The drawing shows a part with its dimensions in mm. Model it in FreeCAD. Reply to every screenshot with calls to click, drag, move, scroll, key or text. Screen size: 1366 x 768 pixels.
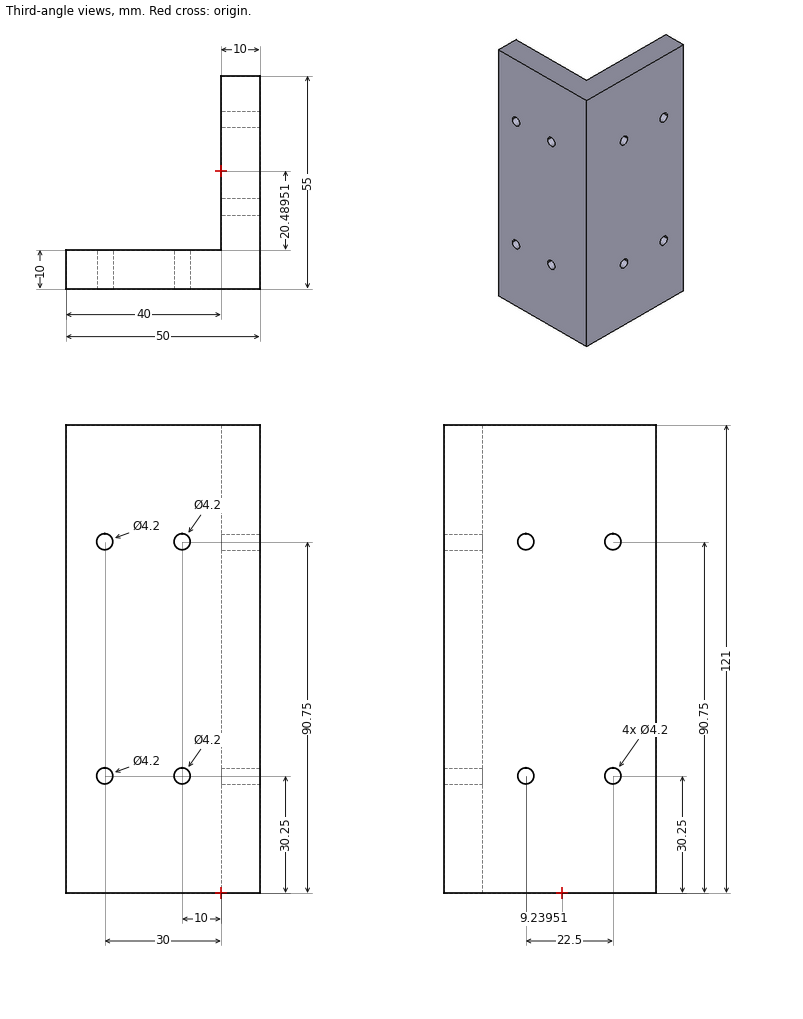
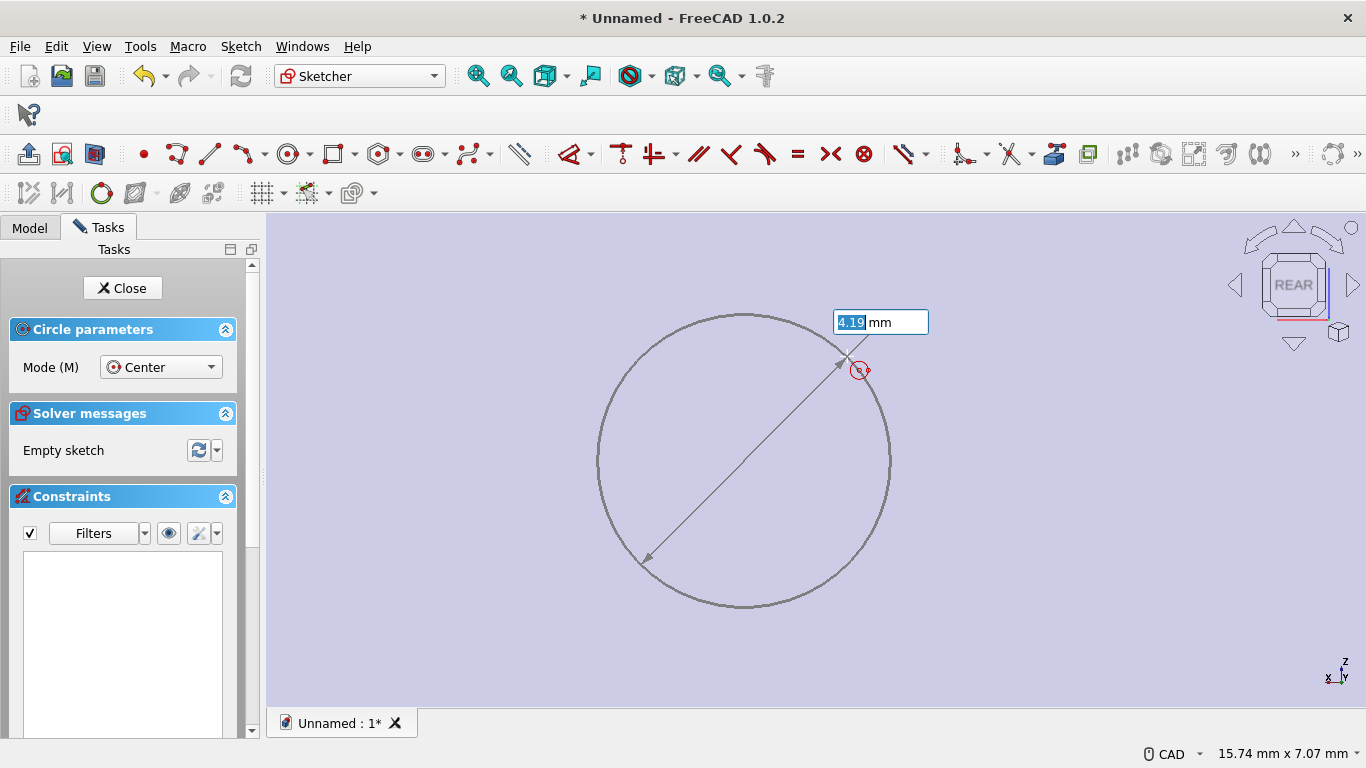
text(4.2)
key(Return)
key(Escape)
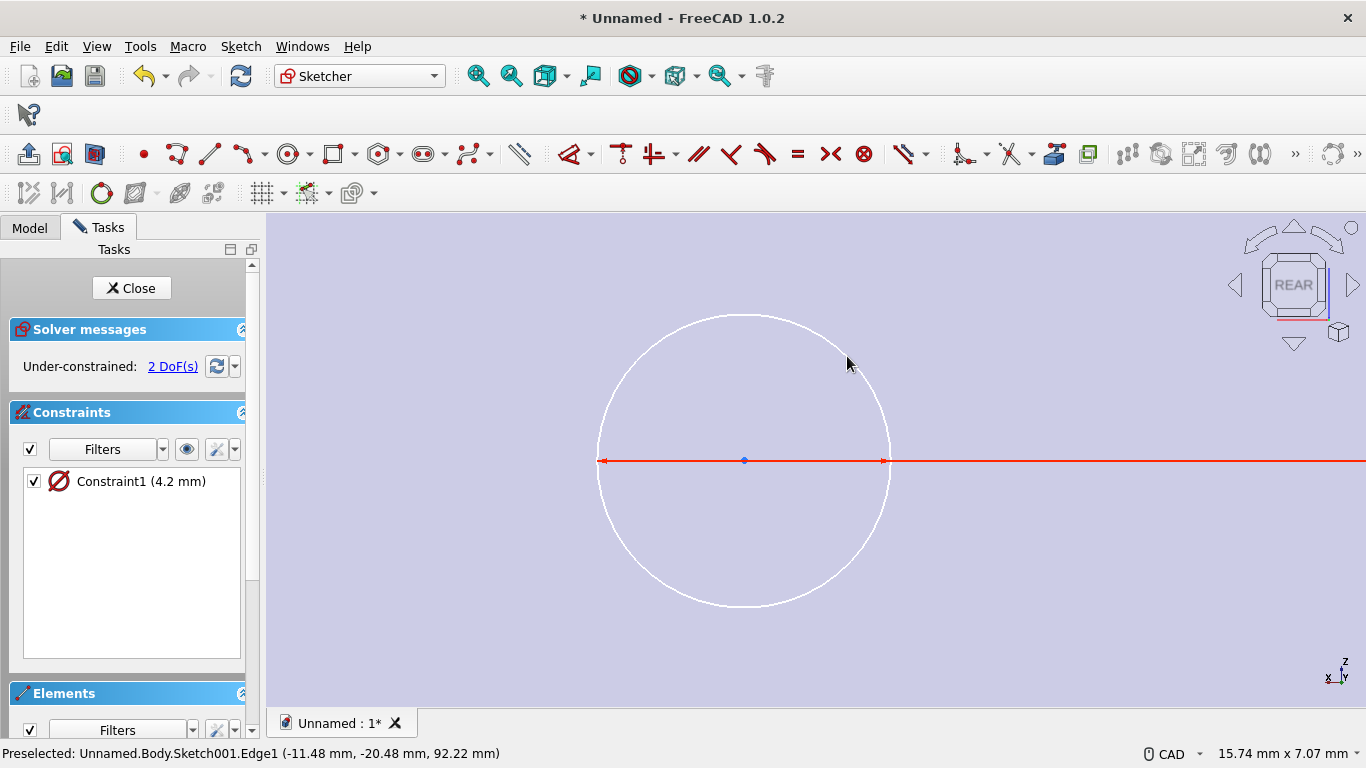
key(d)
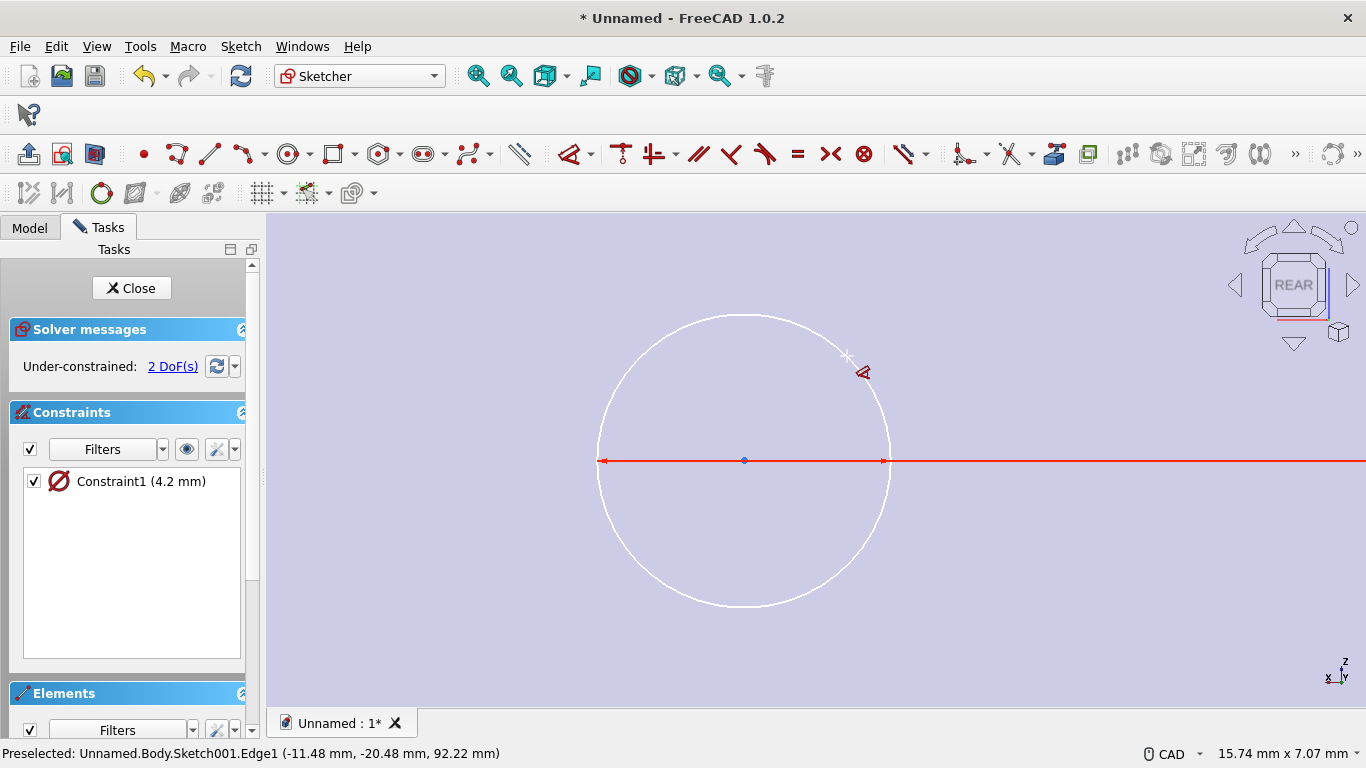
click(744, 461)
click(519, 427)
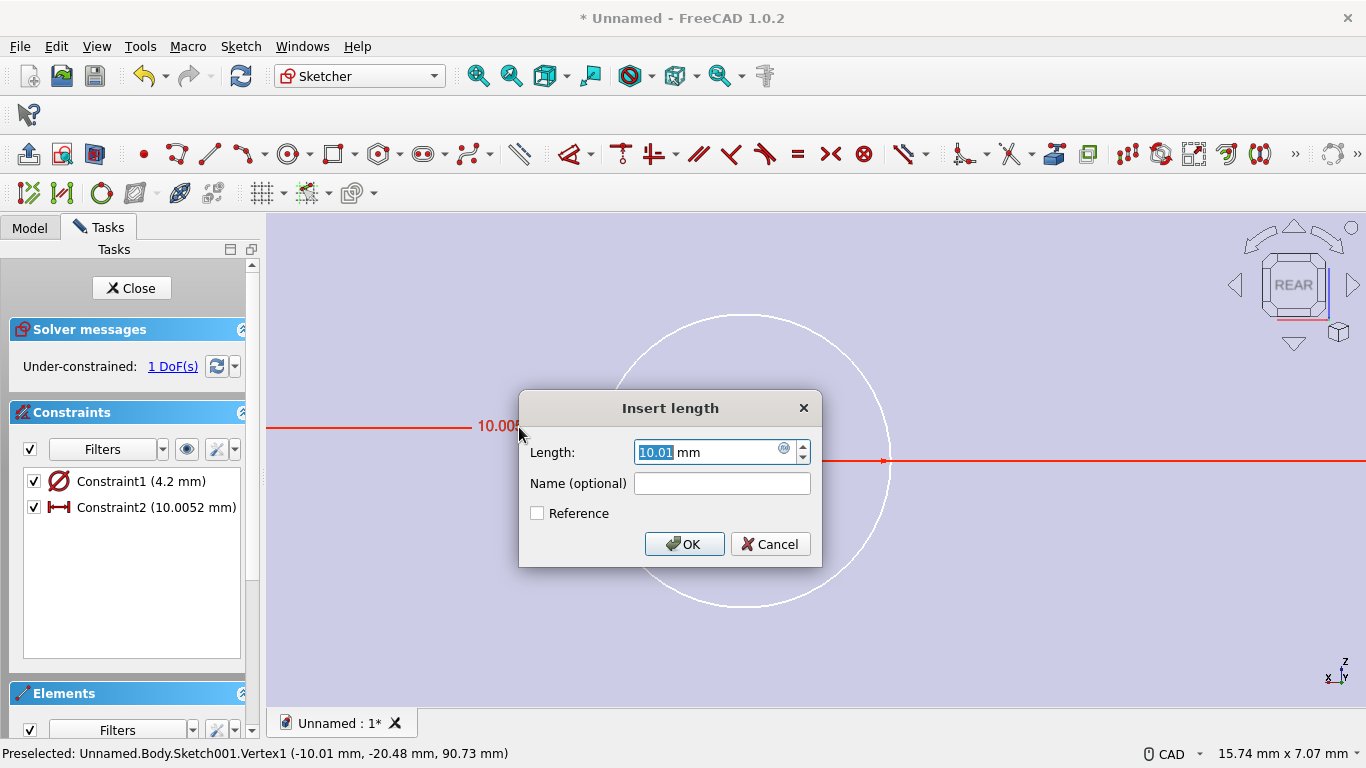
text(10)
key(Return)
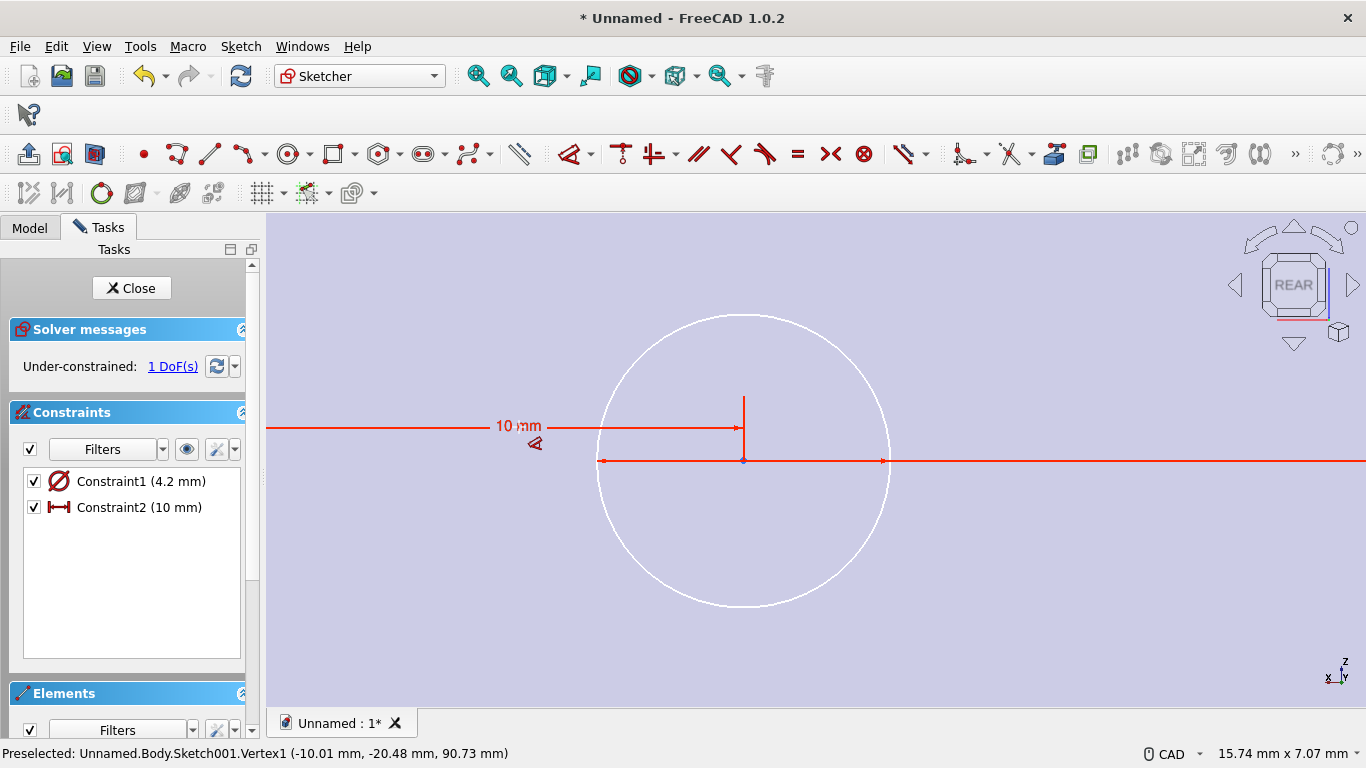
click(744, 461)
click(778, 570)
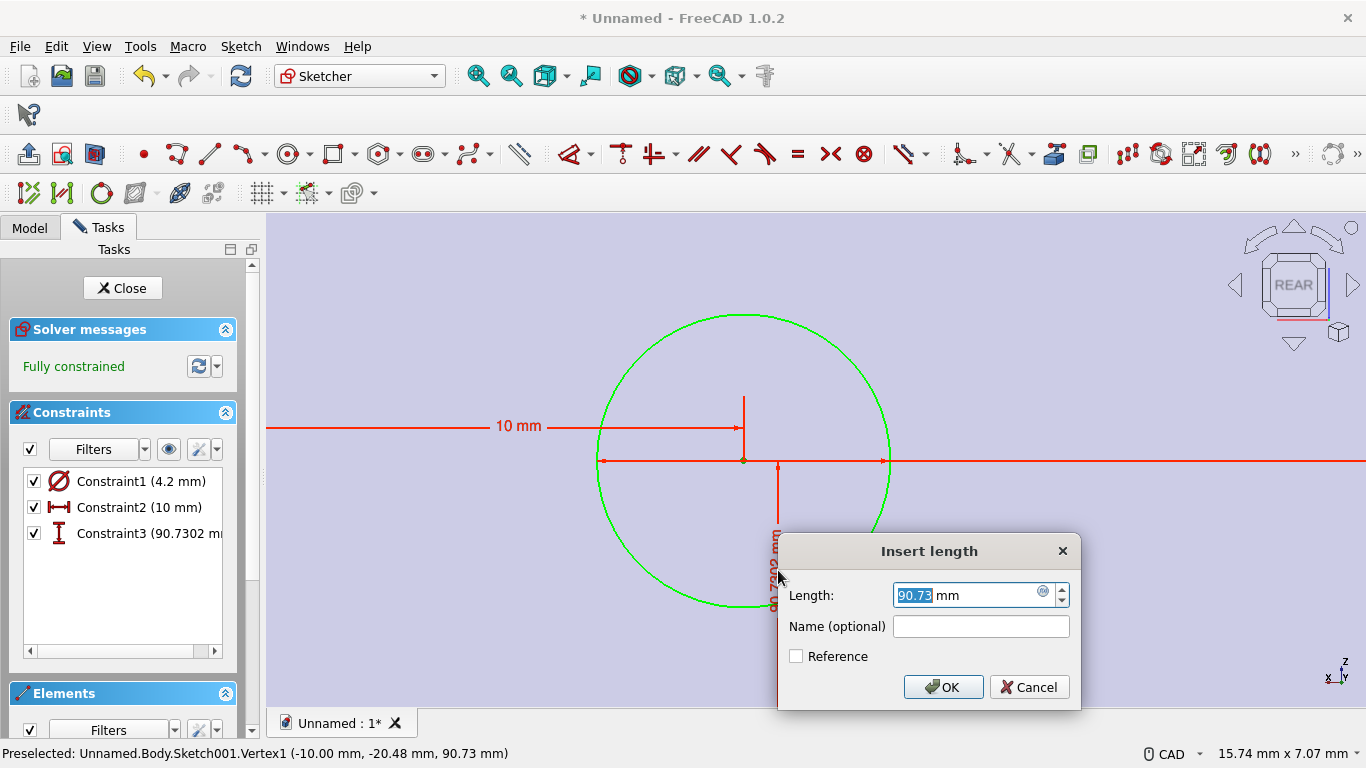
text(90.75)
key(Return)
key(Escape)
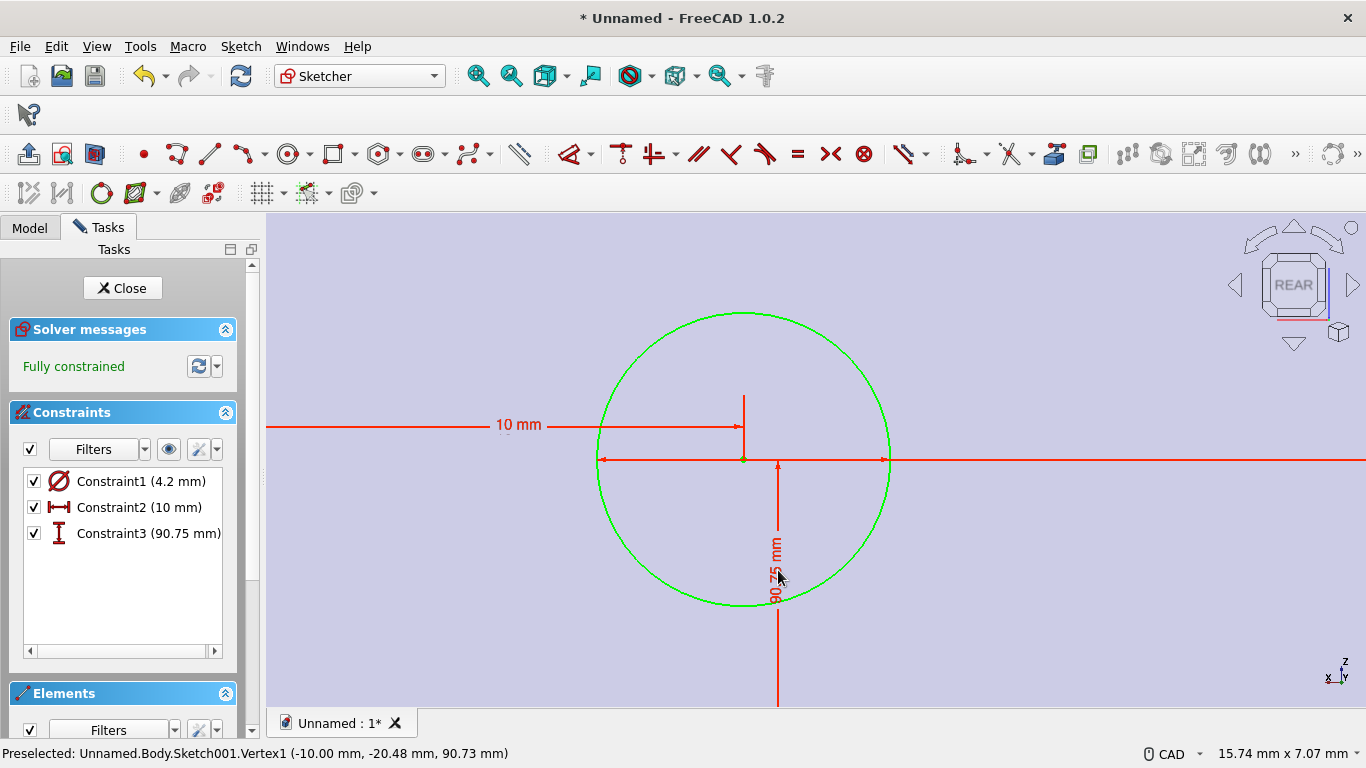
click(123, 288)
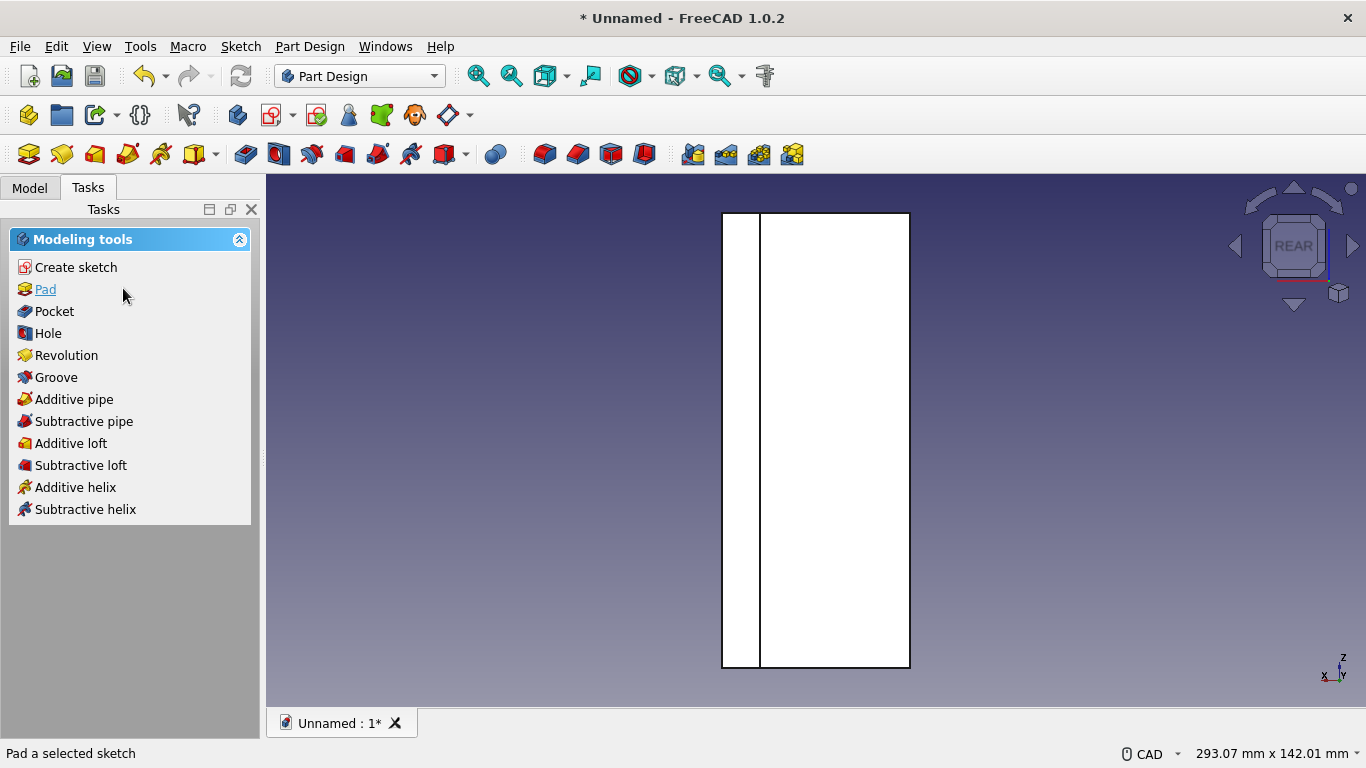
click(246, 154)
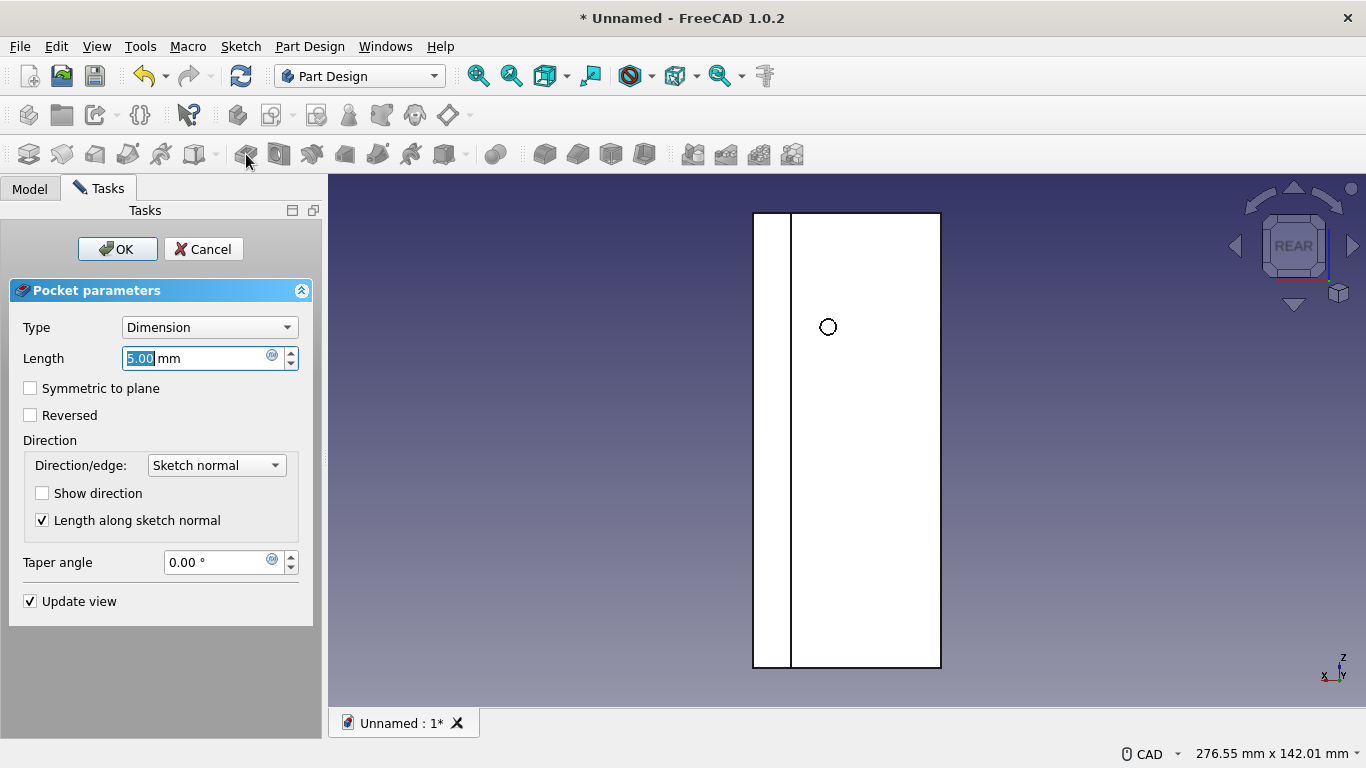
click(210, 328)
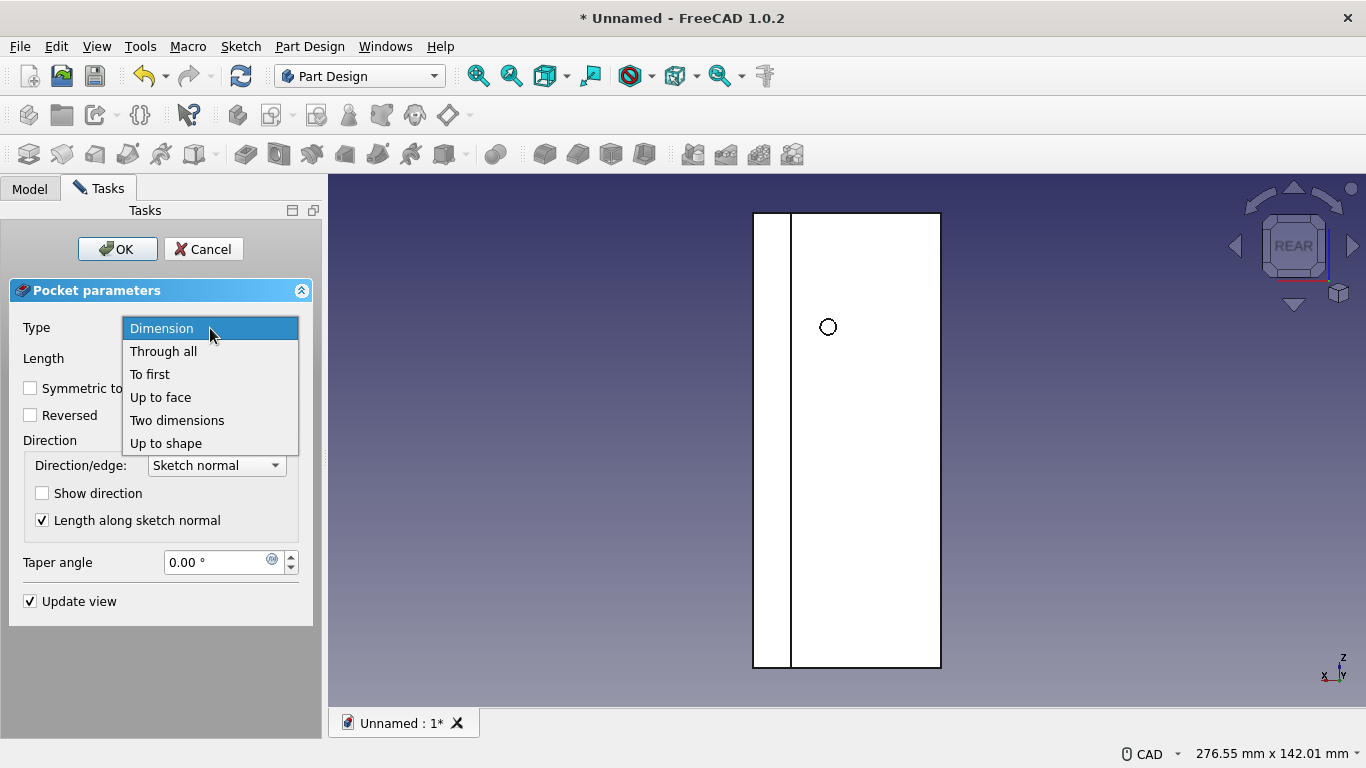
click(208, 374)